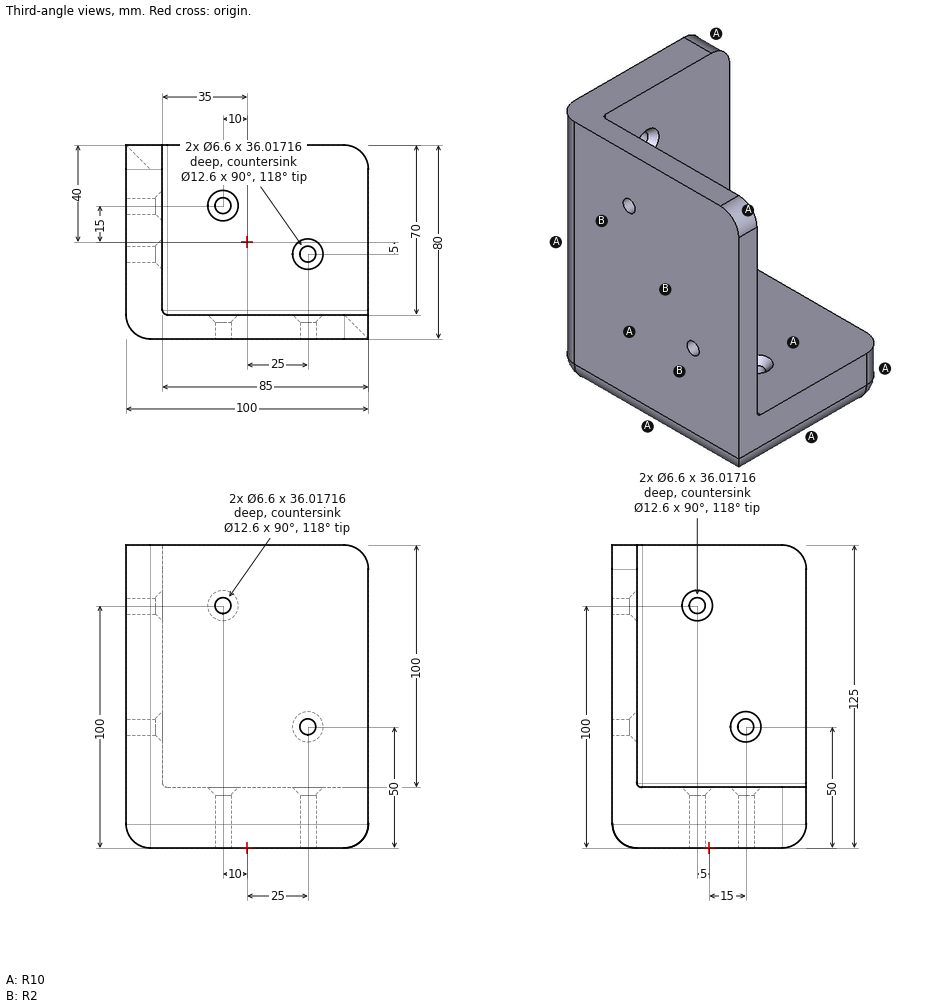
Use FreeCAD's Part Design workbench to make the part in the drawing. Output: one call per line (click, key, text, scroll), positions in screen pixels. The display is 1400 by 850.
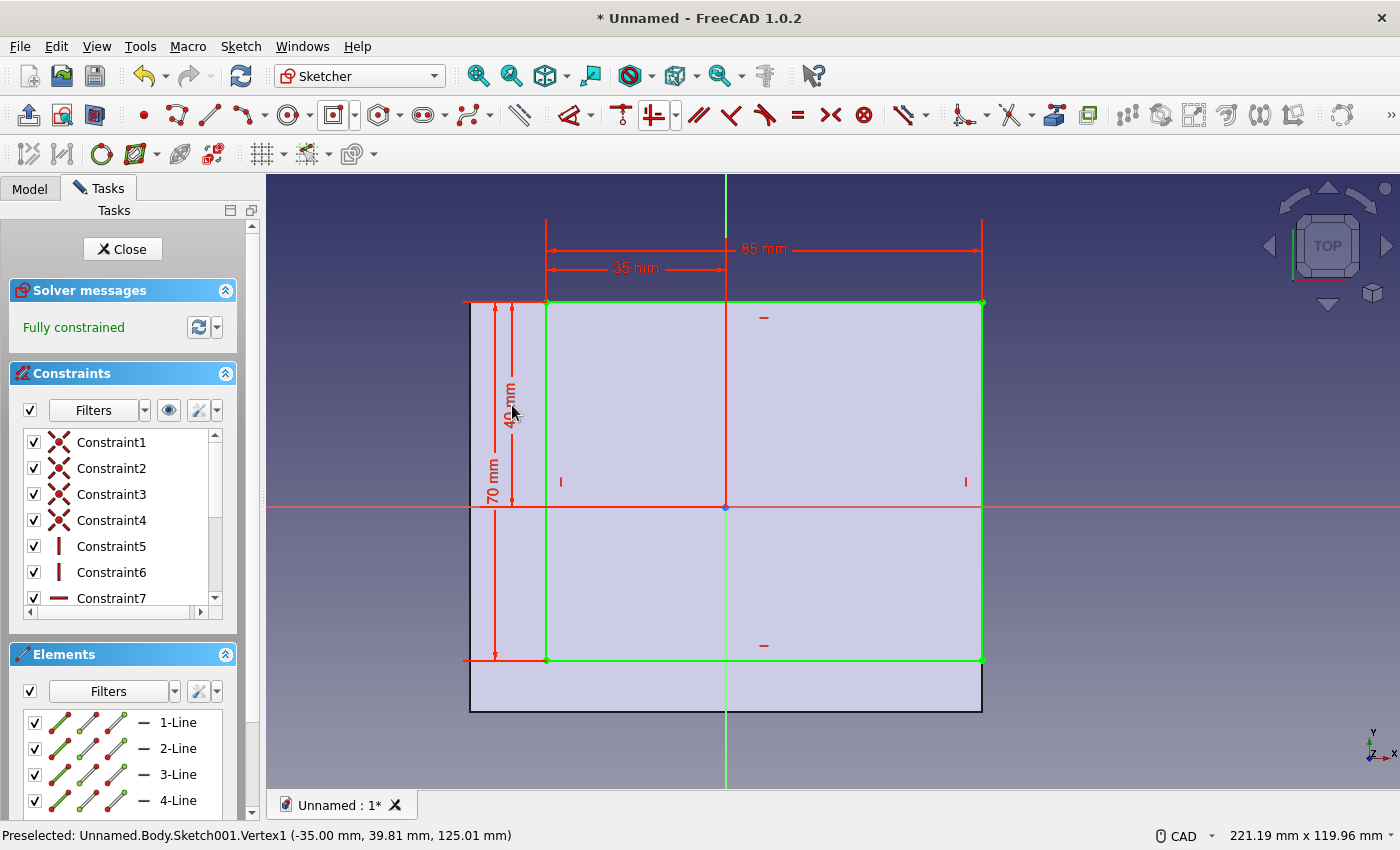
click(123, 249)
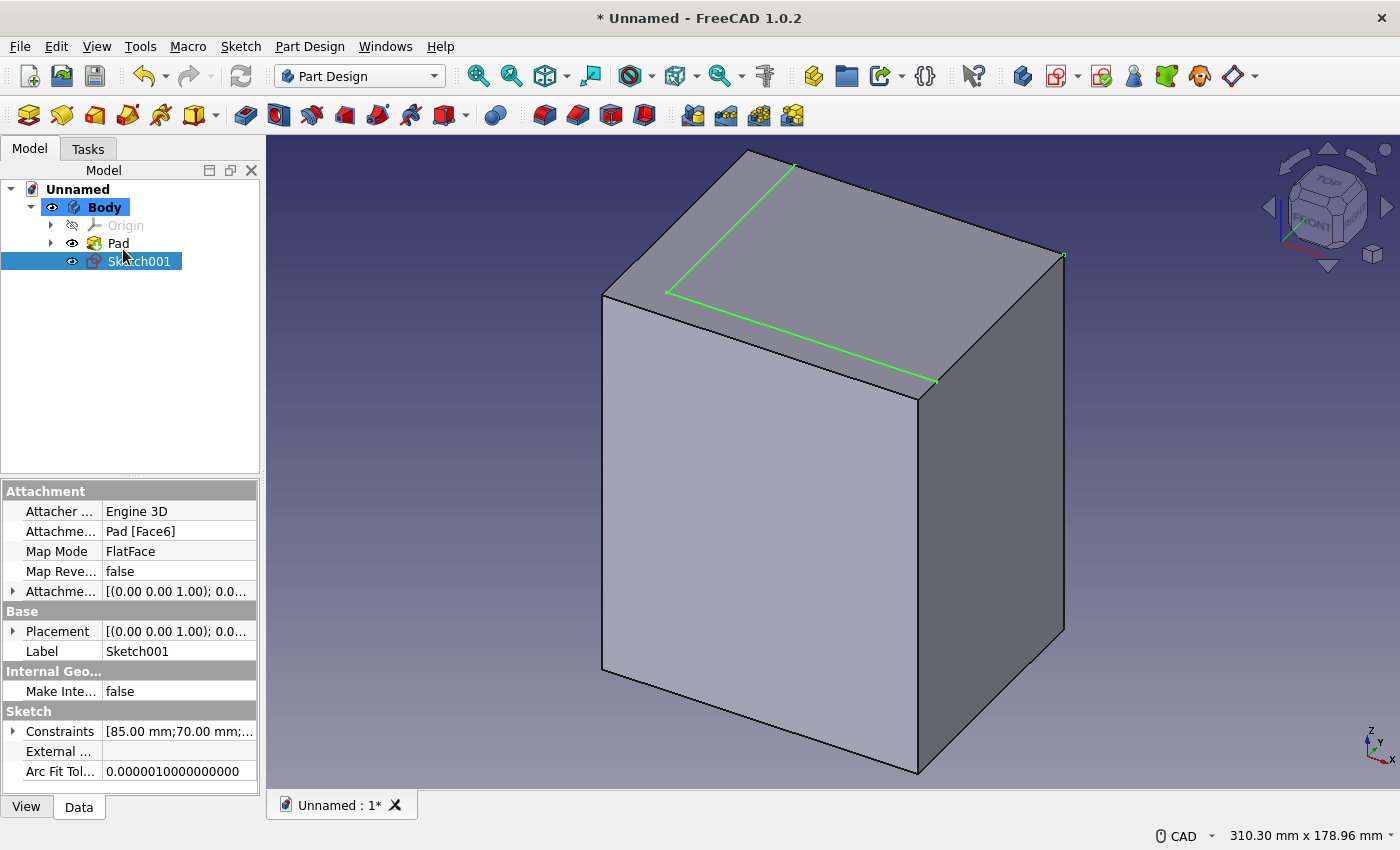
click(246, 116)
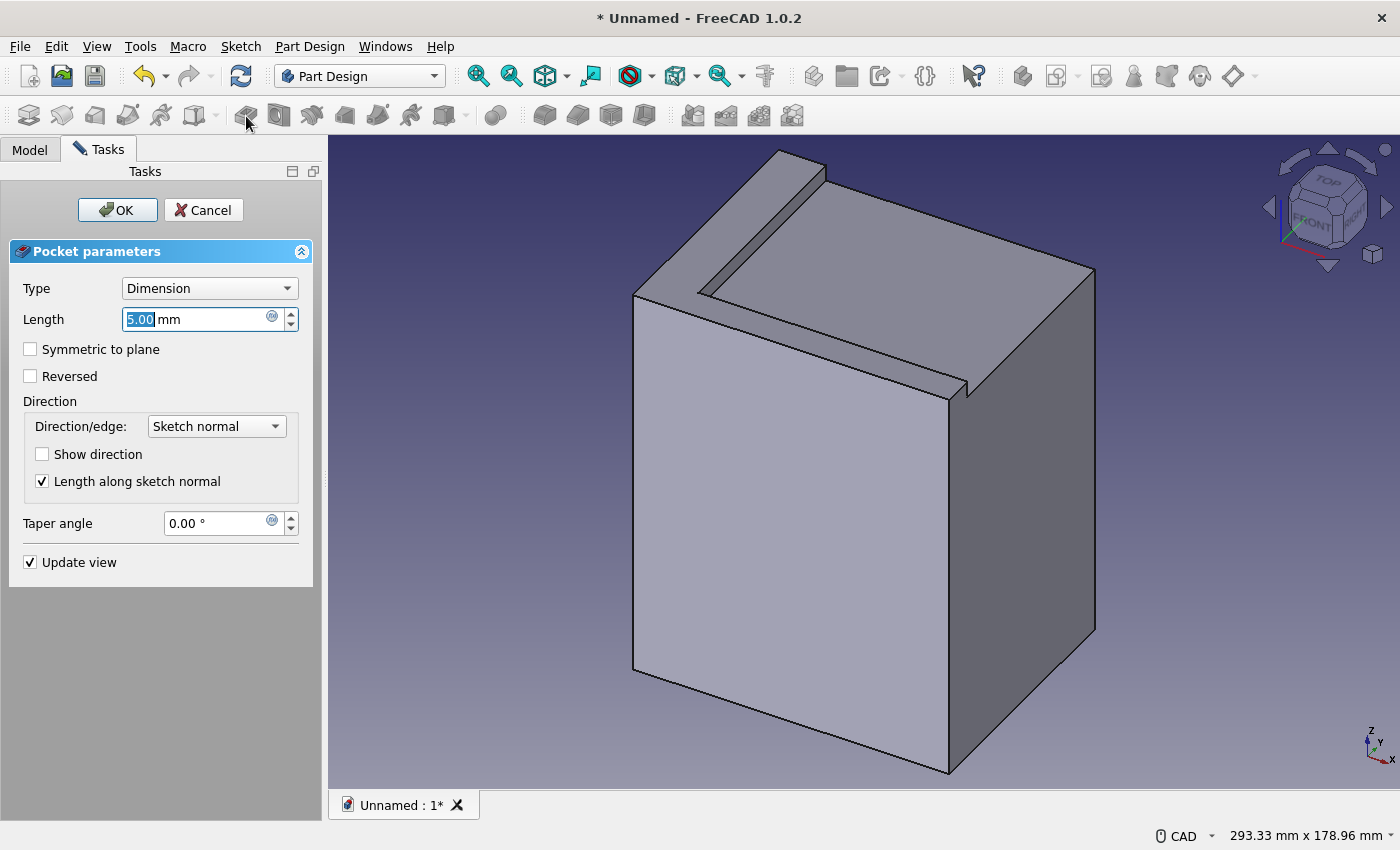
text(100)
key(Tab)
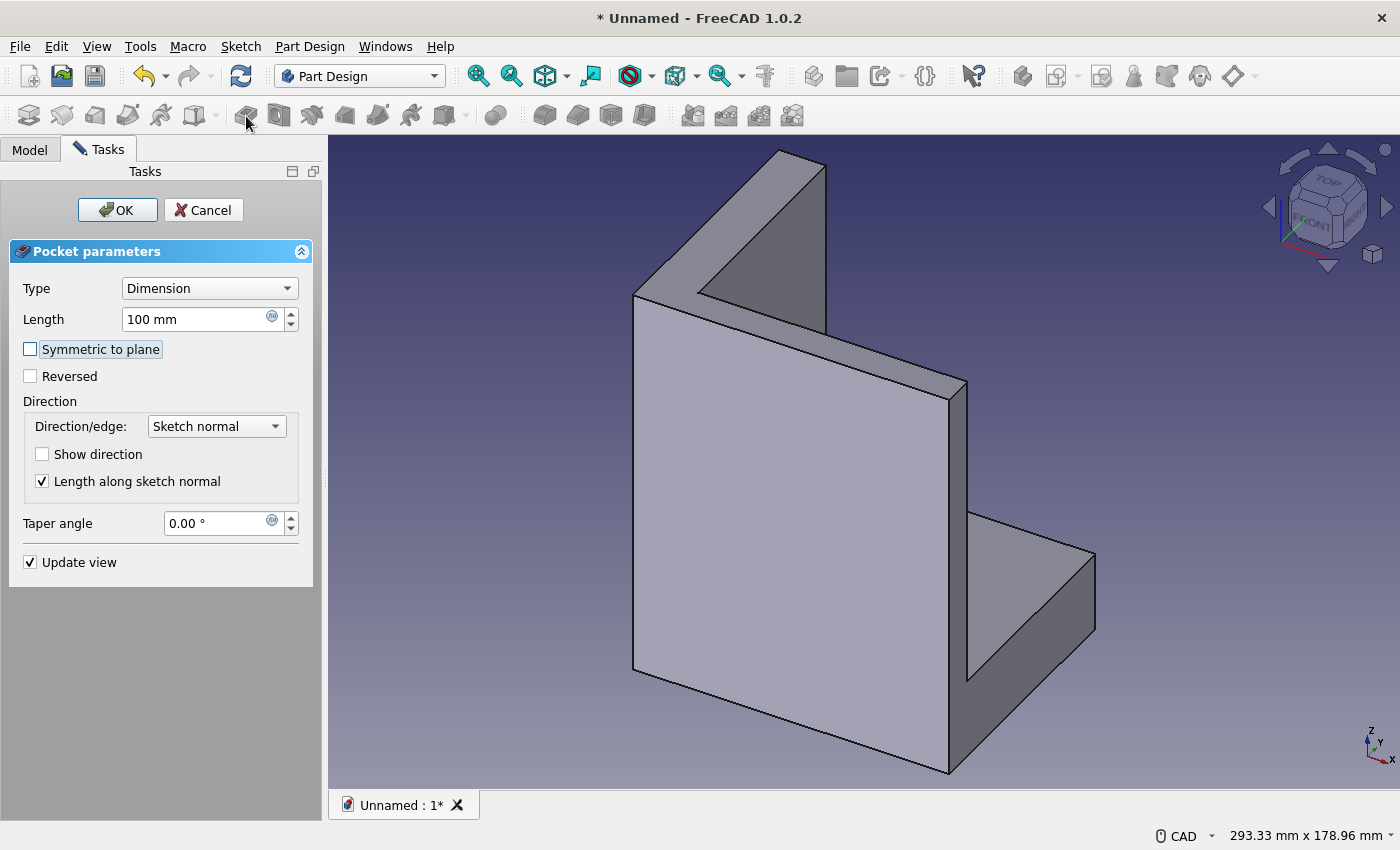
click(118, 210)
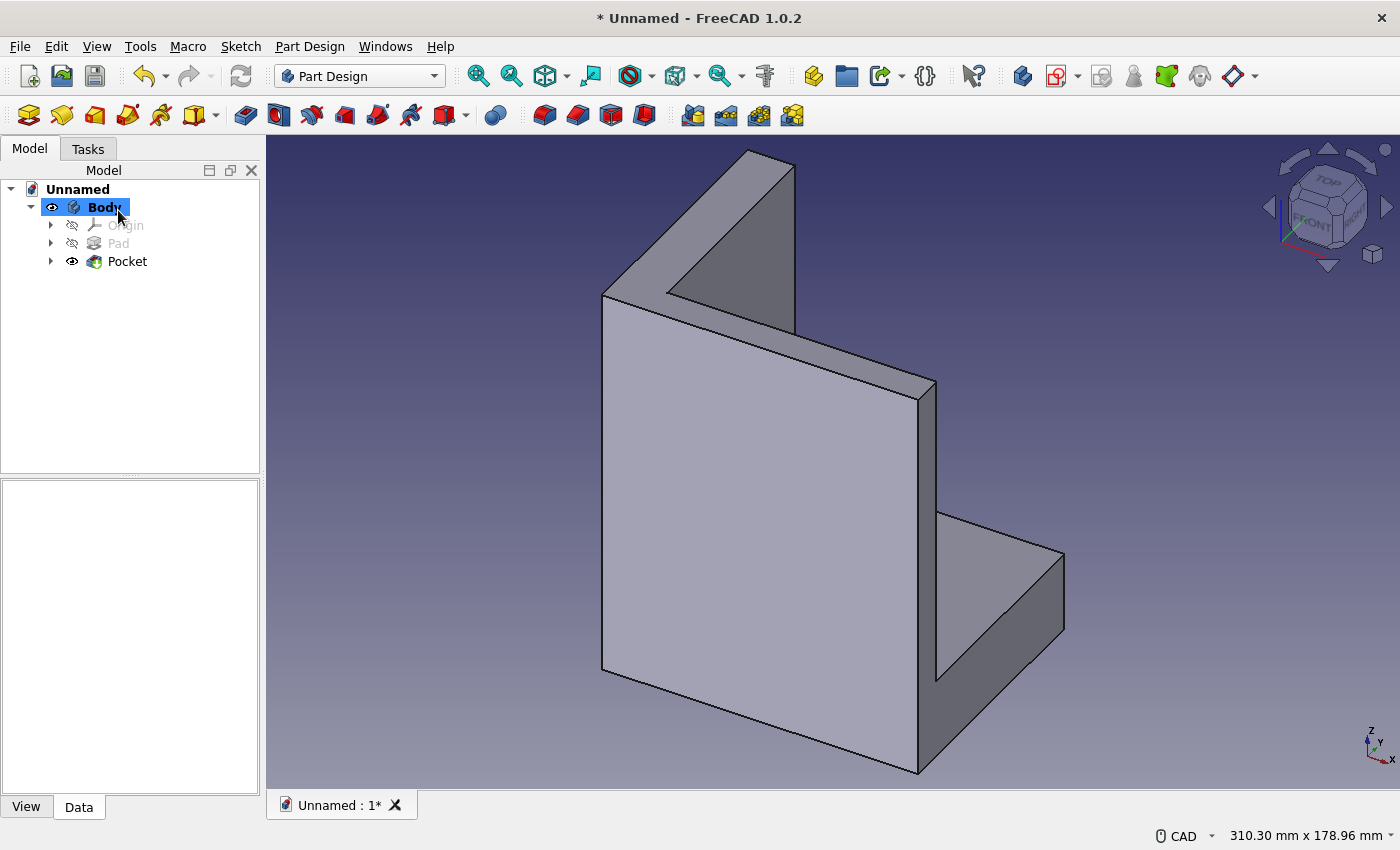
key(0)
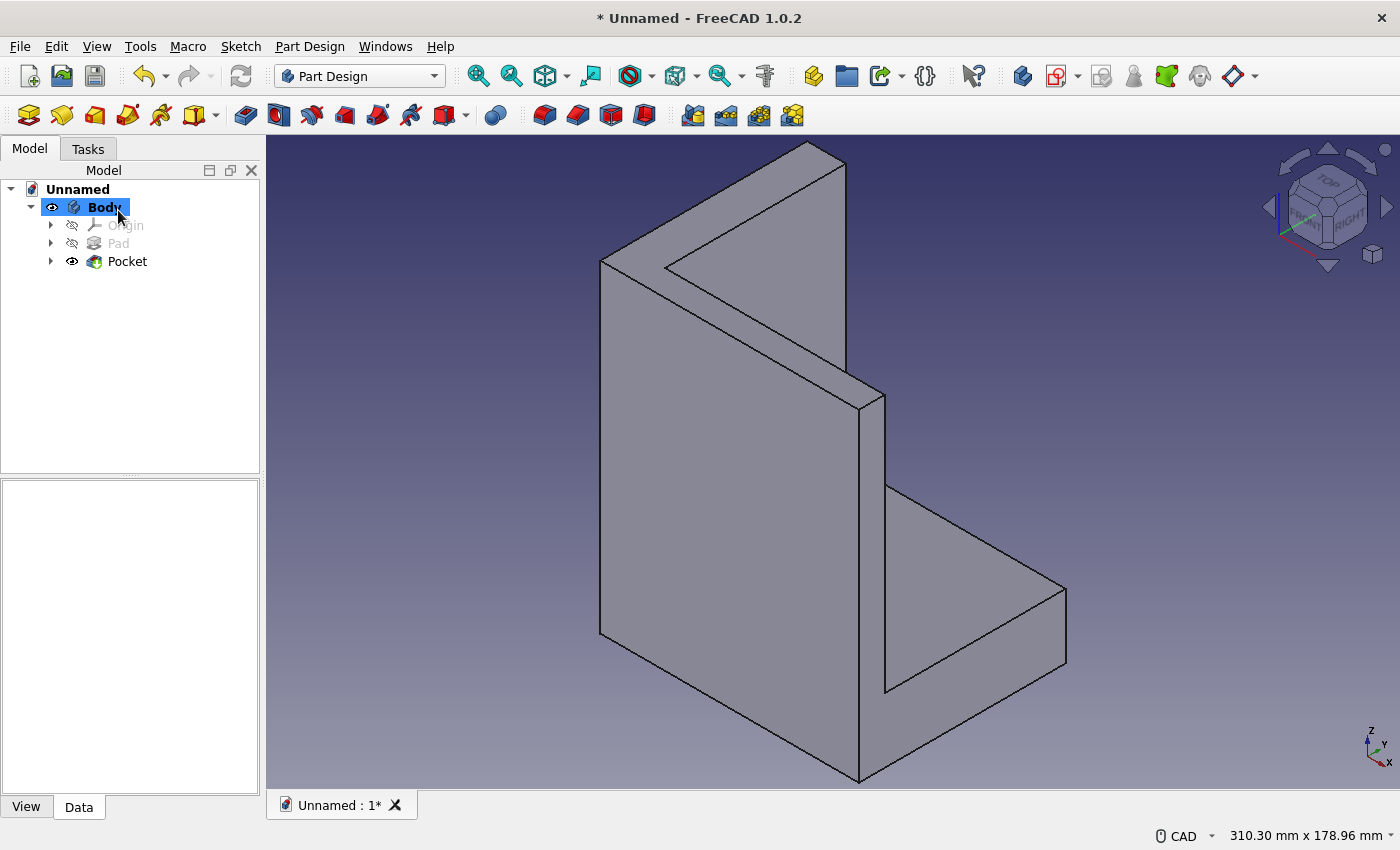
click(781, 306)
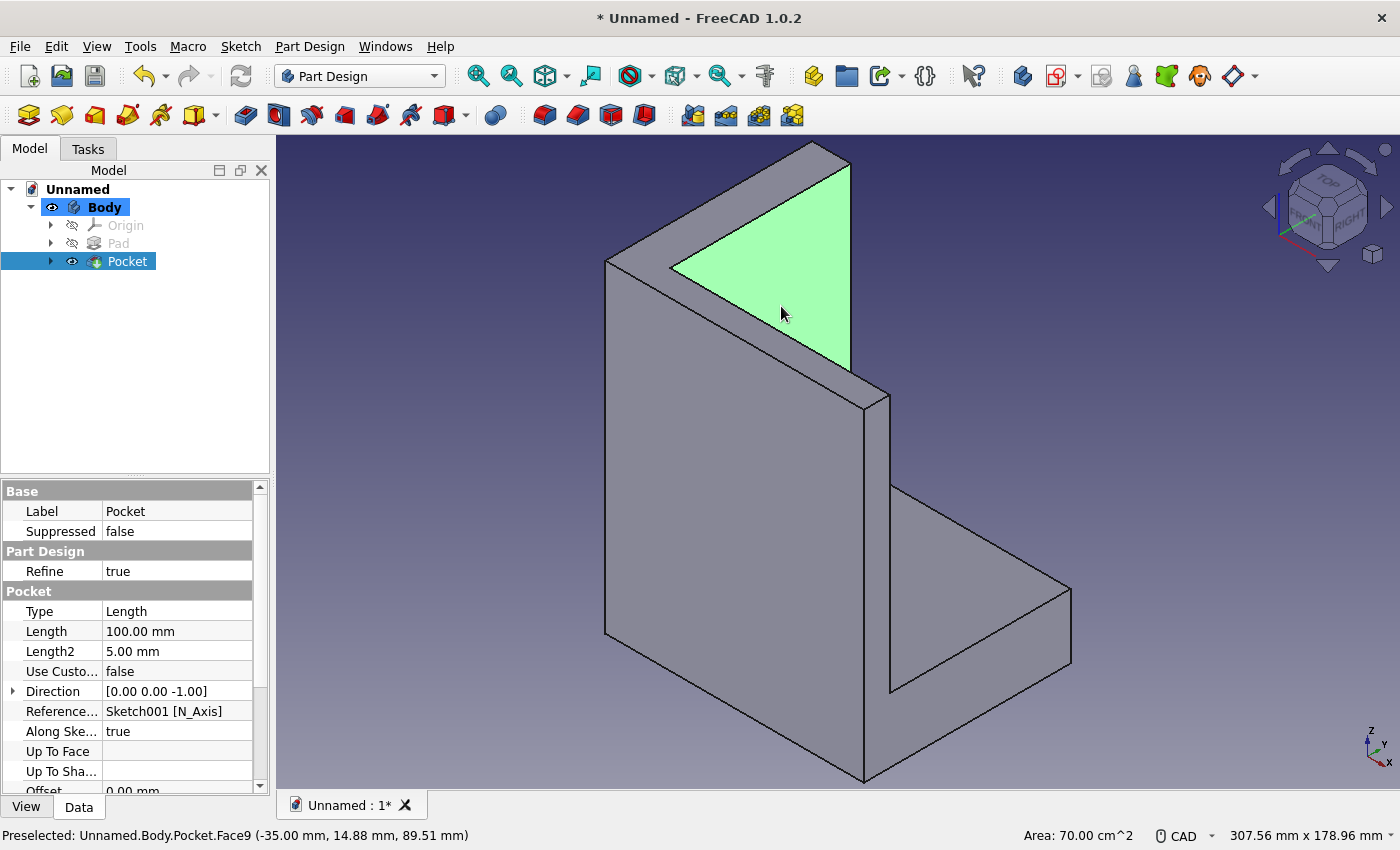
click(1056, 76)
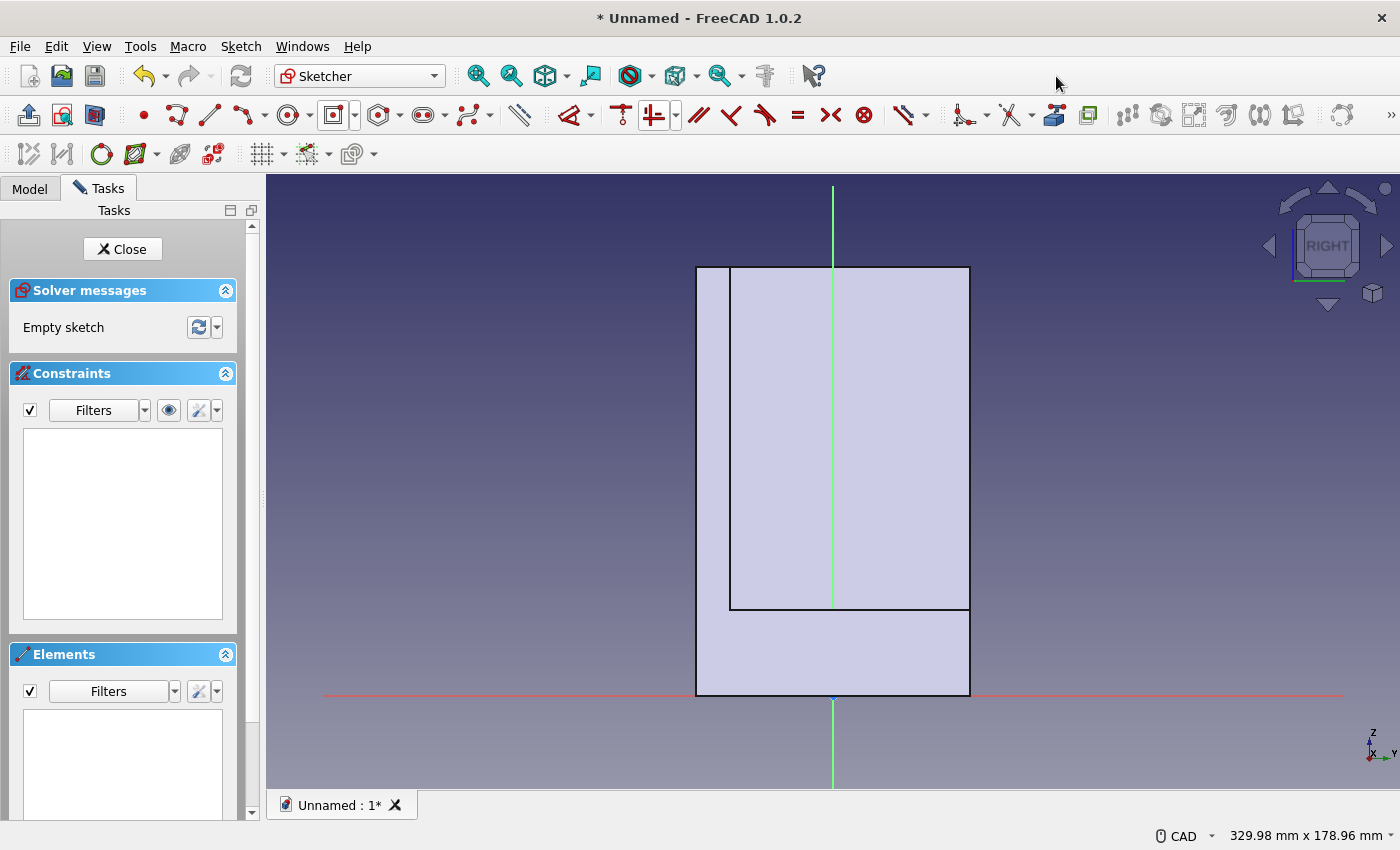
click(95, 116)